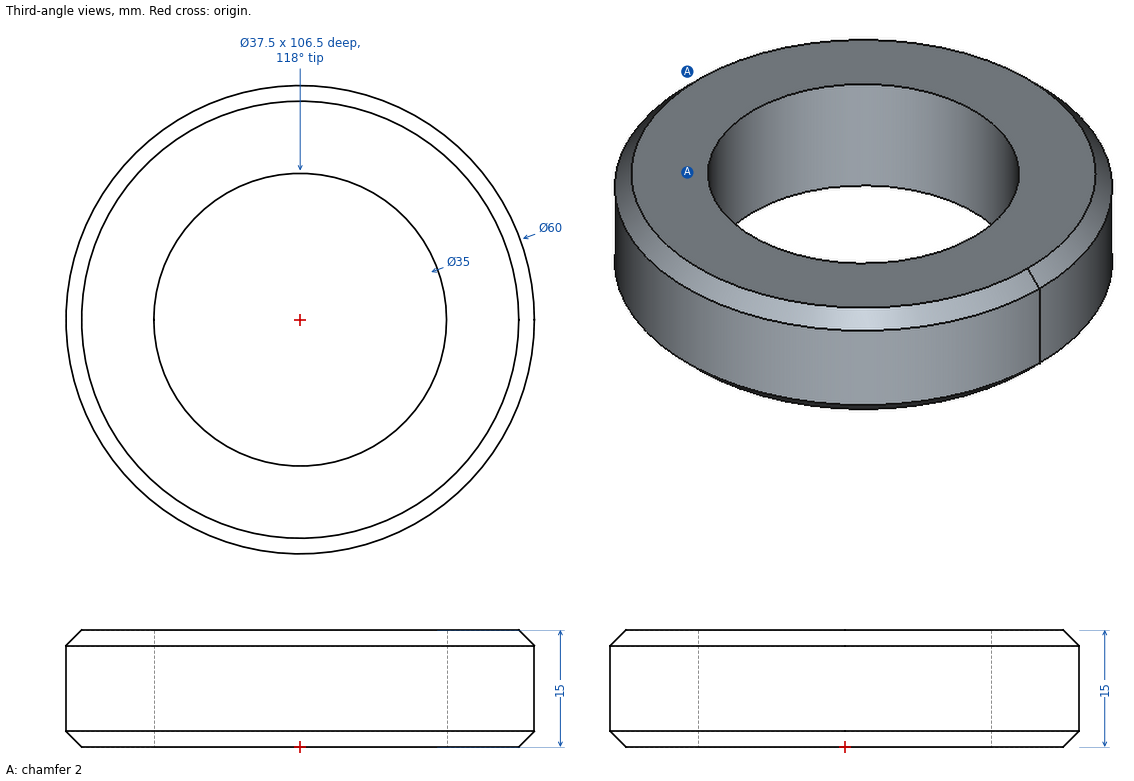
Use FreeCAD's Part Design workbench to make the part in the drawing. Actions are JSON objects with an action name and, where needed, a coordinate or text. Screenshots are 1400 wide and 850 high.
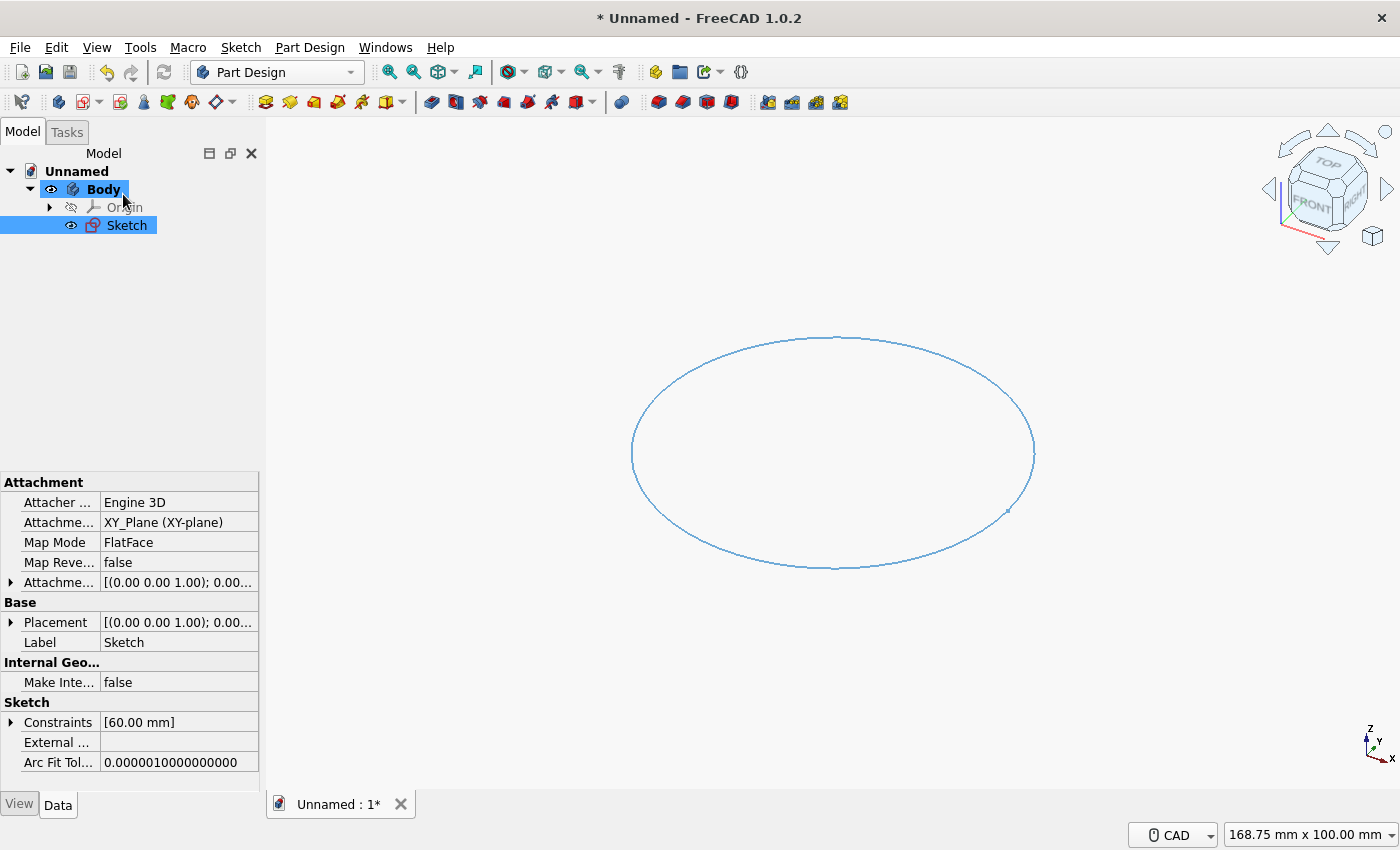
{"action": "left_click", "coordinate": [266, 102]}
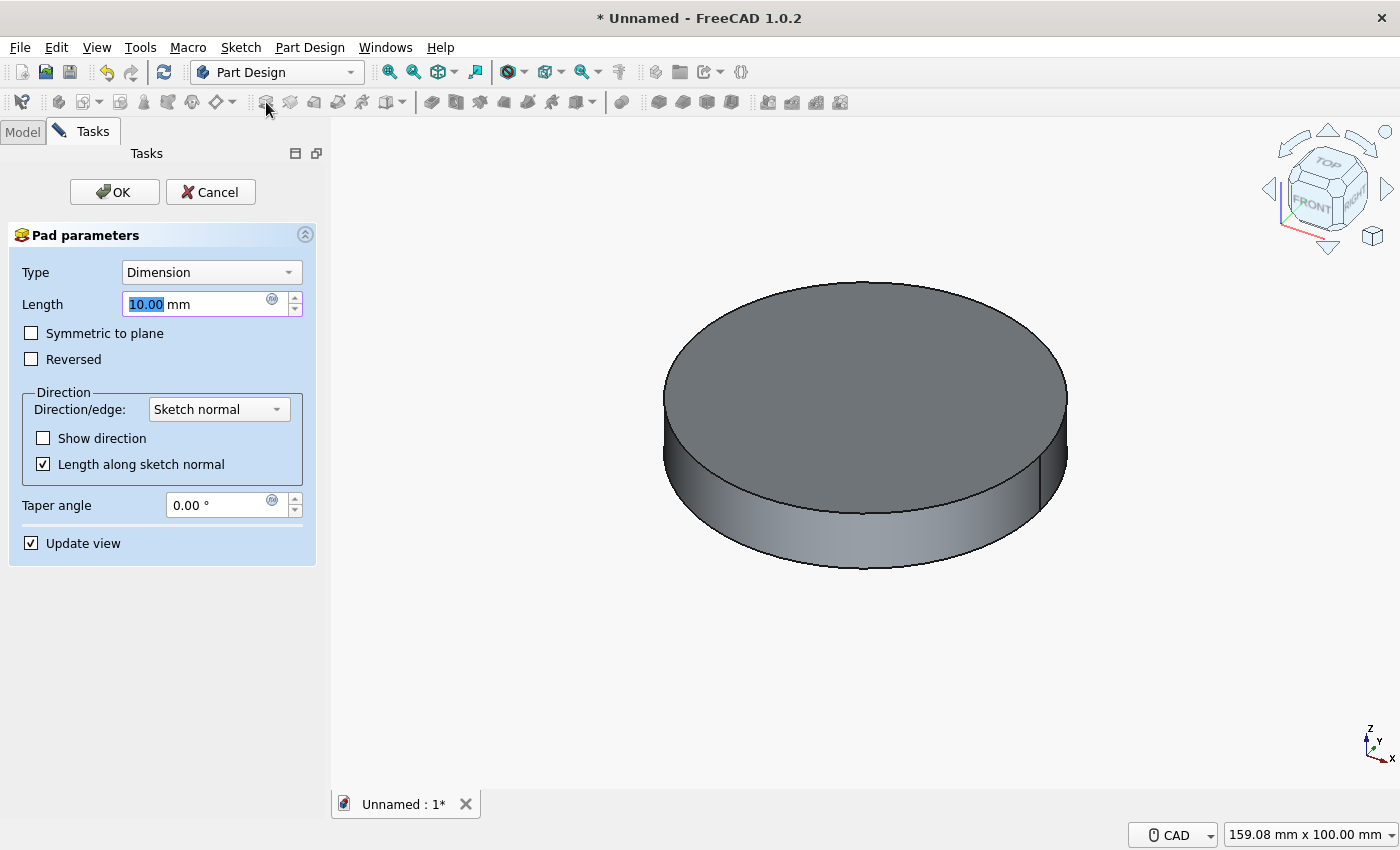
{"action": "type", "text": "15"}
{"action": "key", "text": "Tab"}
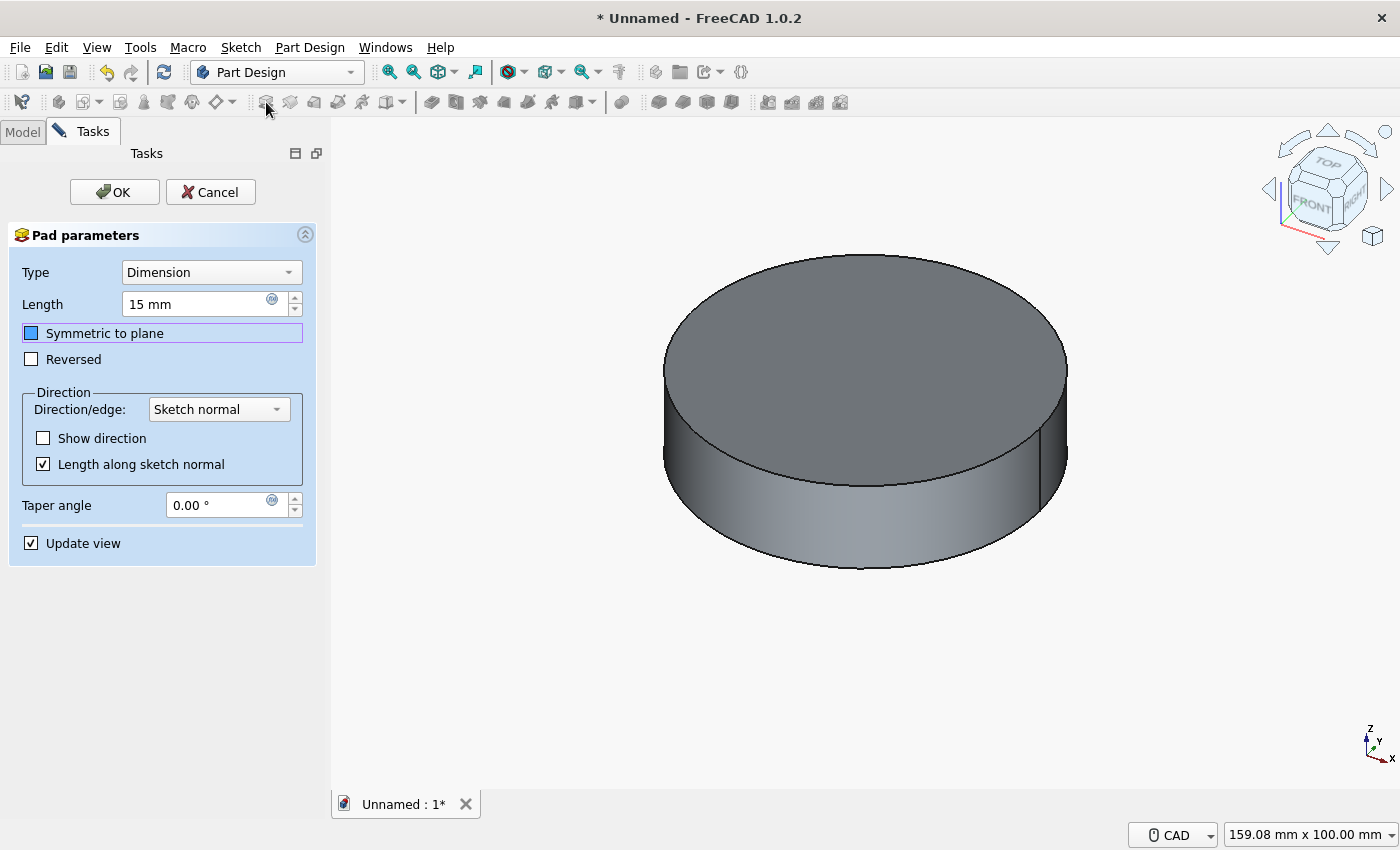
{"action": "left_click", "coordinate": [115, 192]}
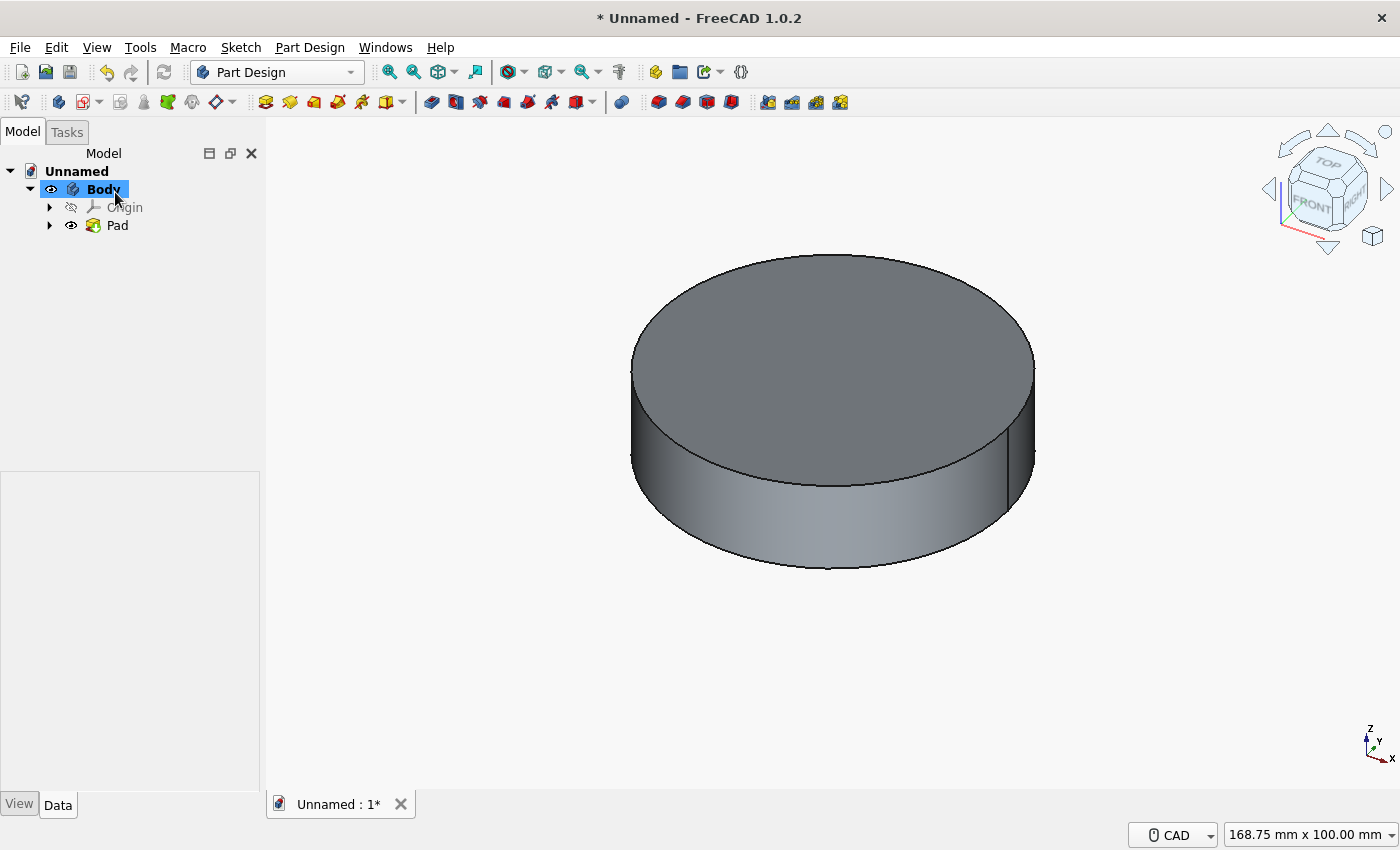
{"action": "left_click", "coordinate": [833, 369]}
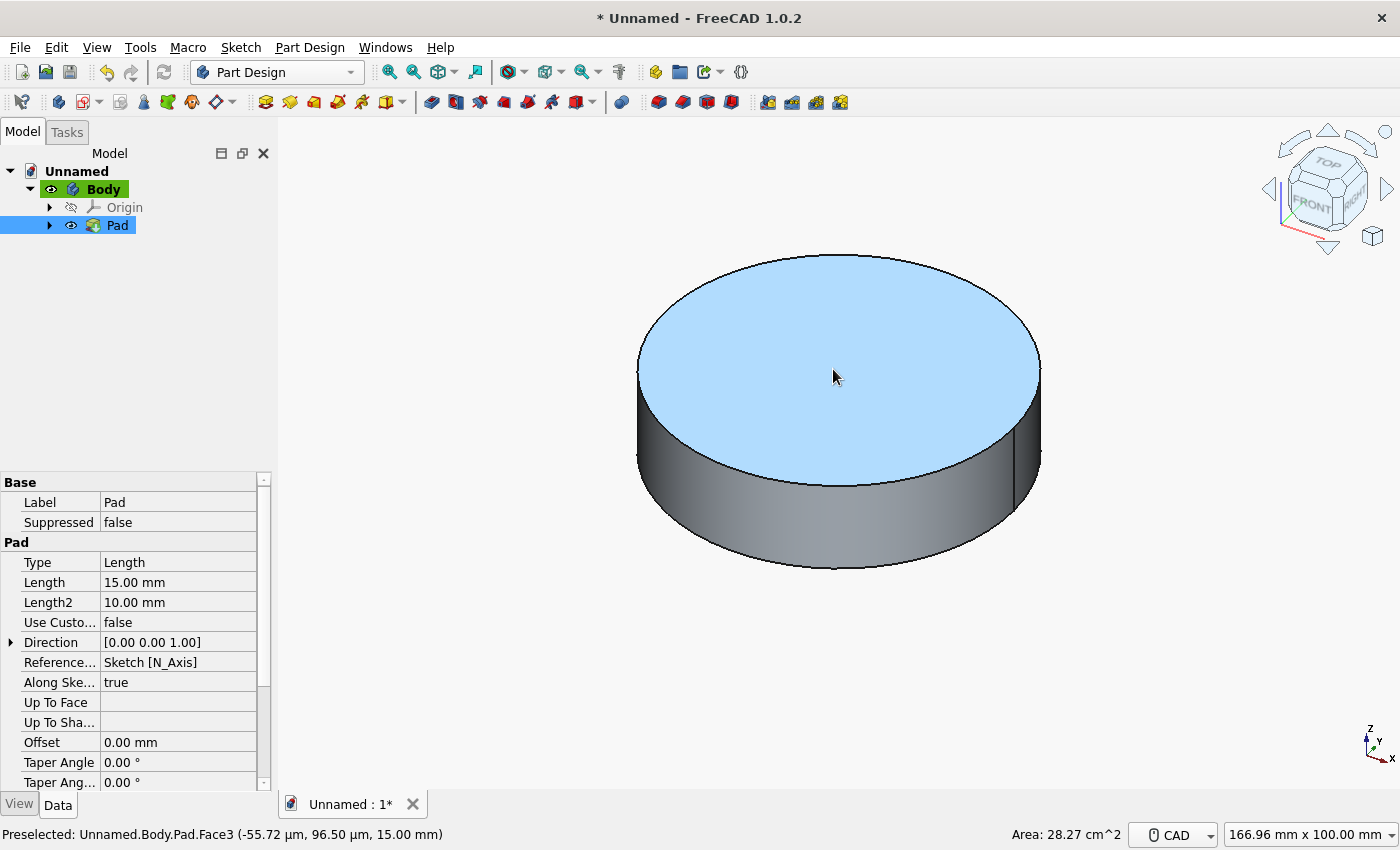
{"action": "left_click", "coordinate": [84, 102]}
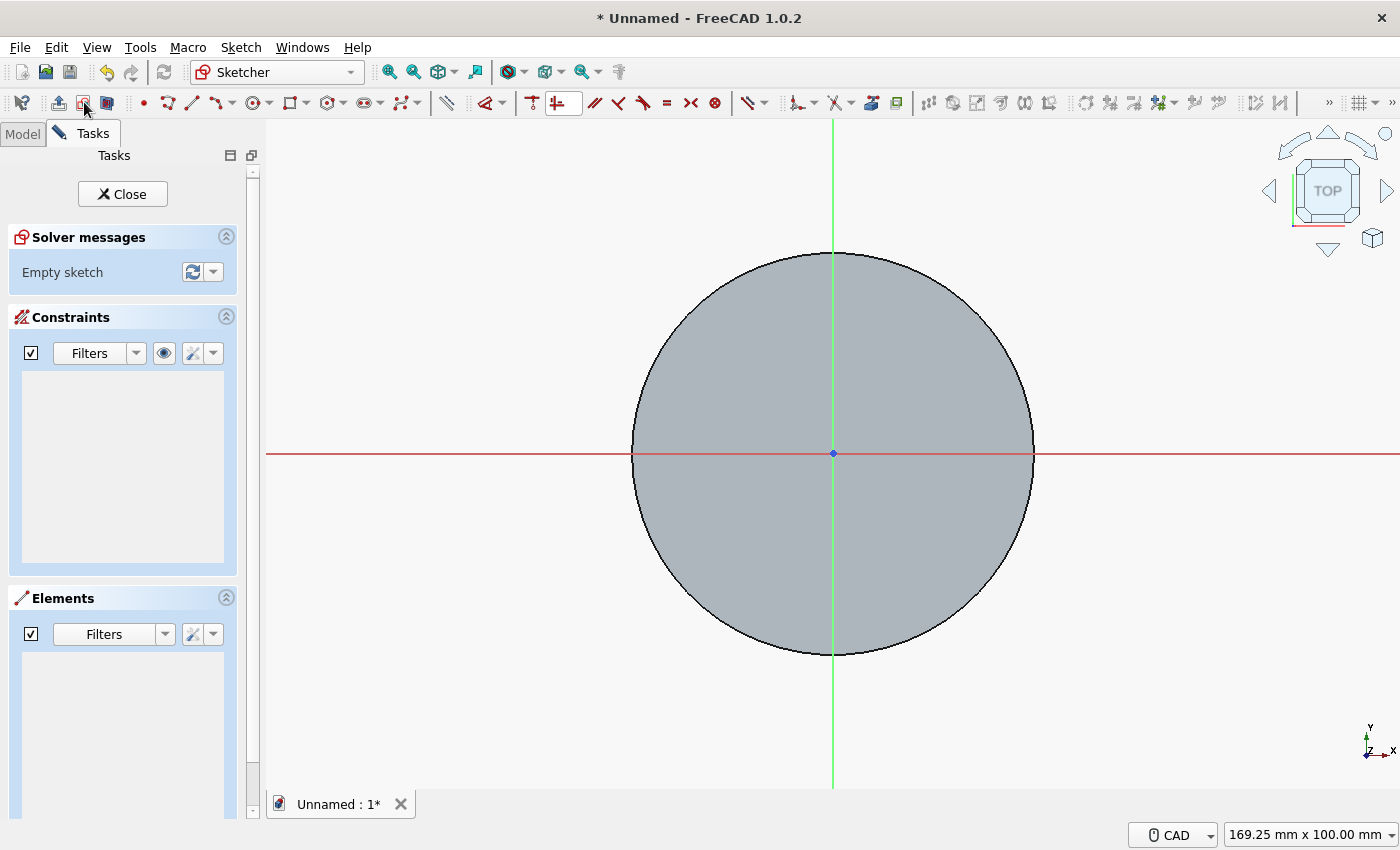
{"action": "scroll", "coordinate": [916, 454], "scroll_direction": "up", "scroll_amount": 3}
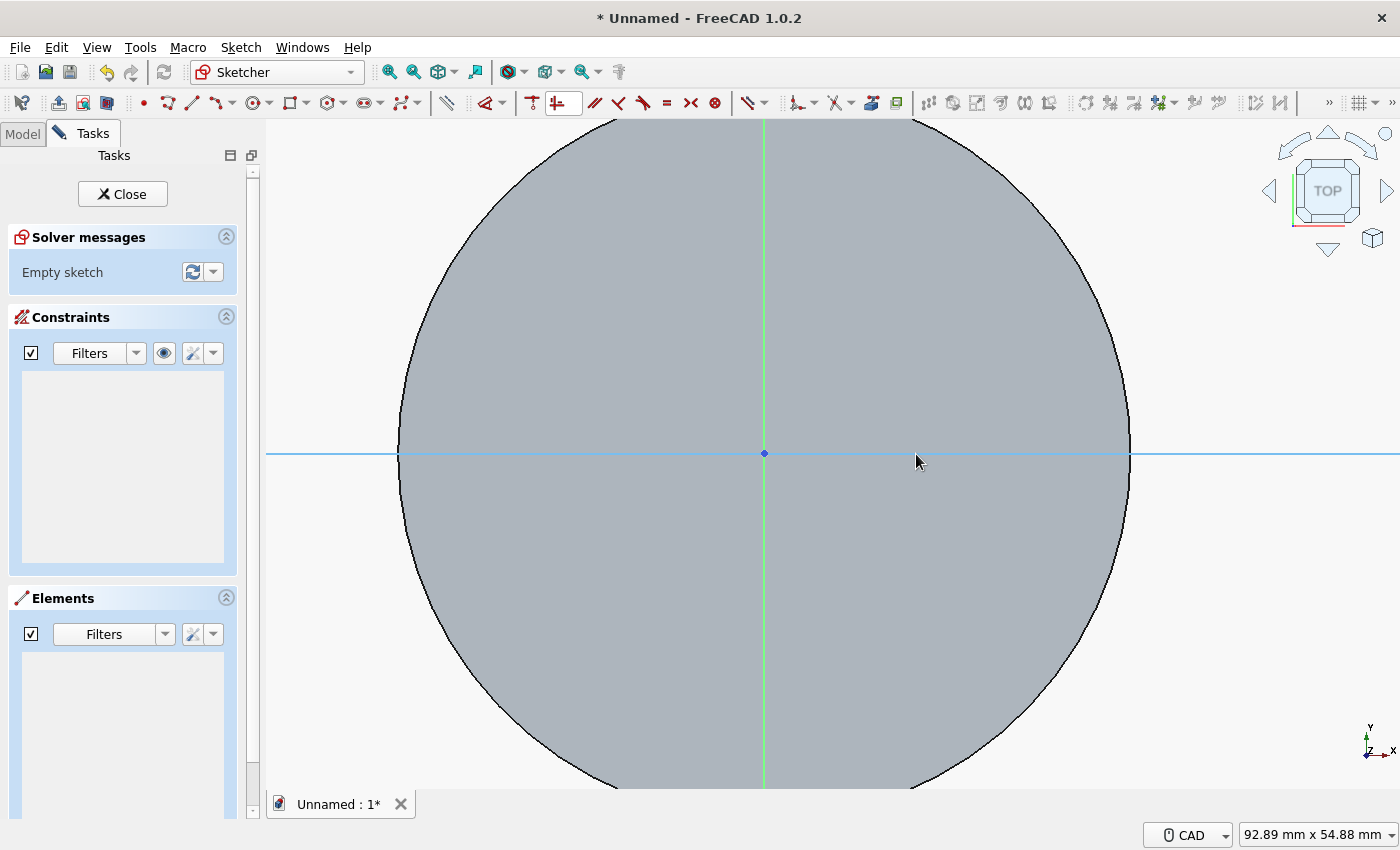
{"action": "left_click", "coordinate": [254, 104]}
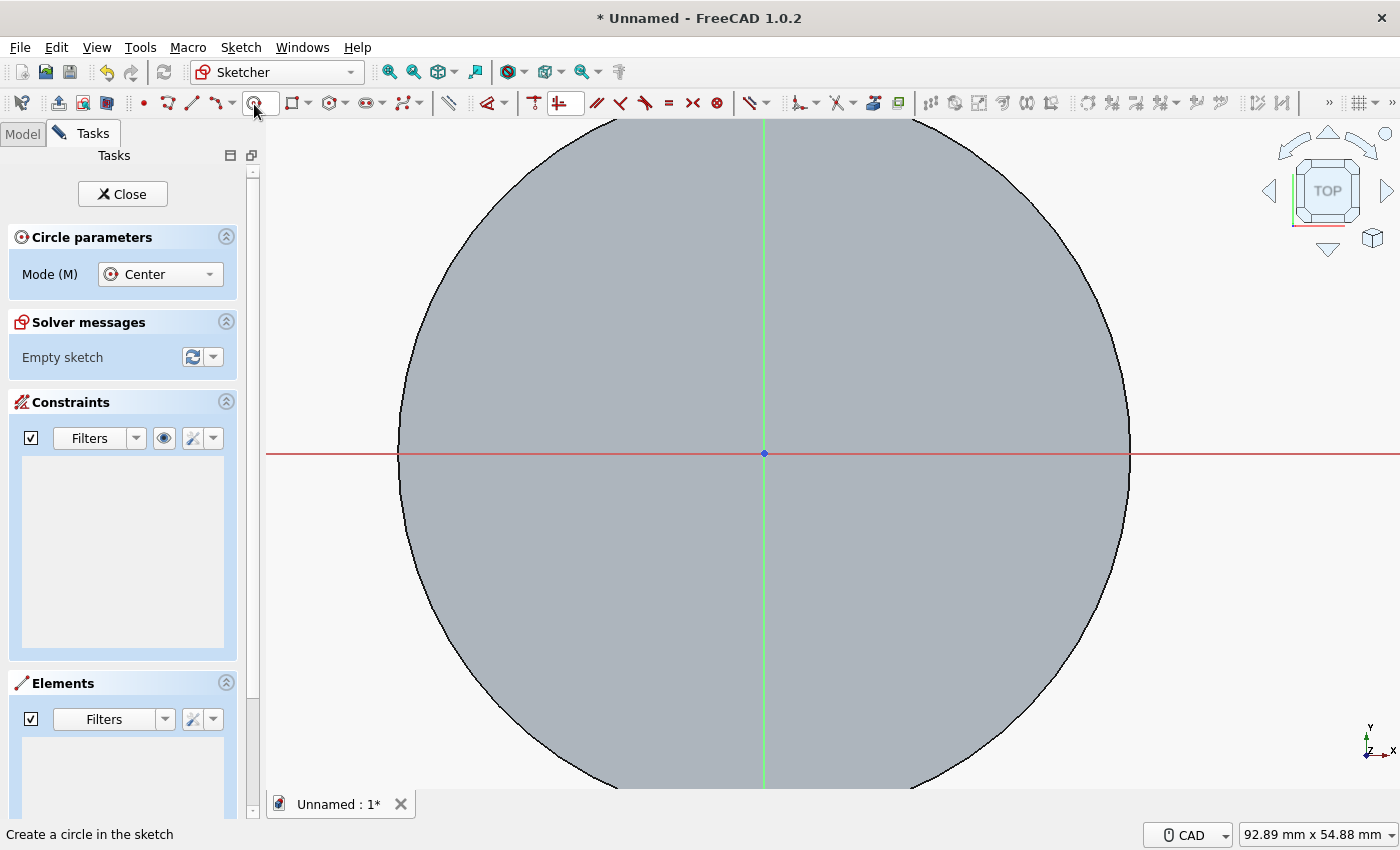
{"action": "left_click", "coordinate": [764, 454]}
{"action": "mouse_move", "coordinate": [915, 303]}